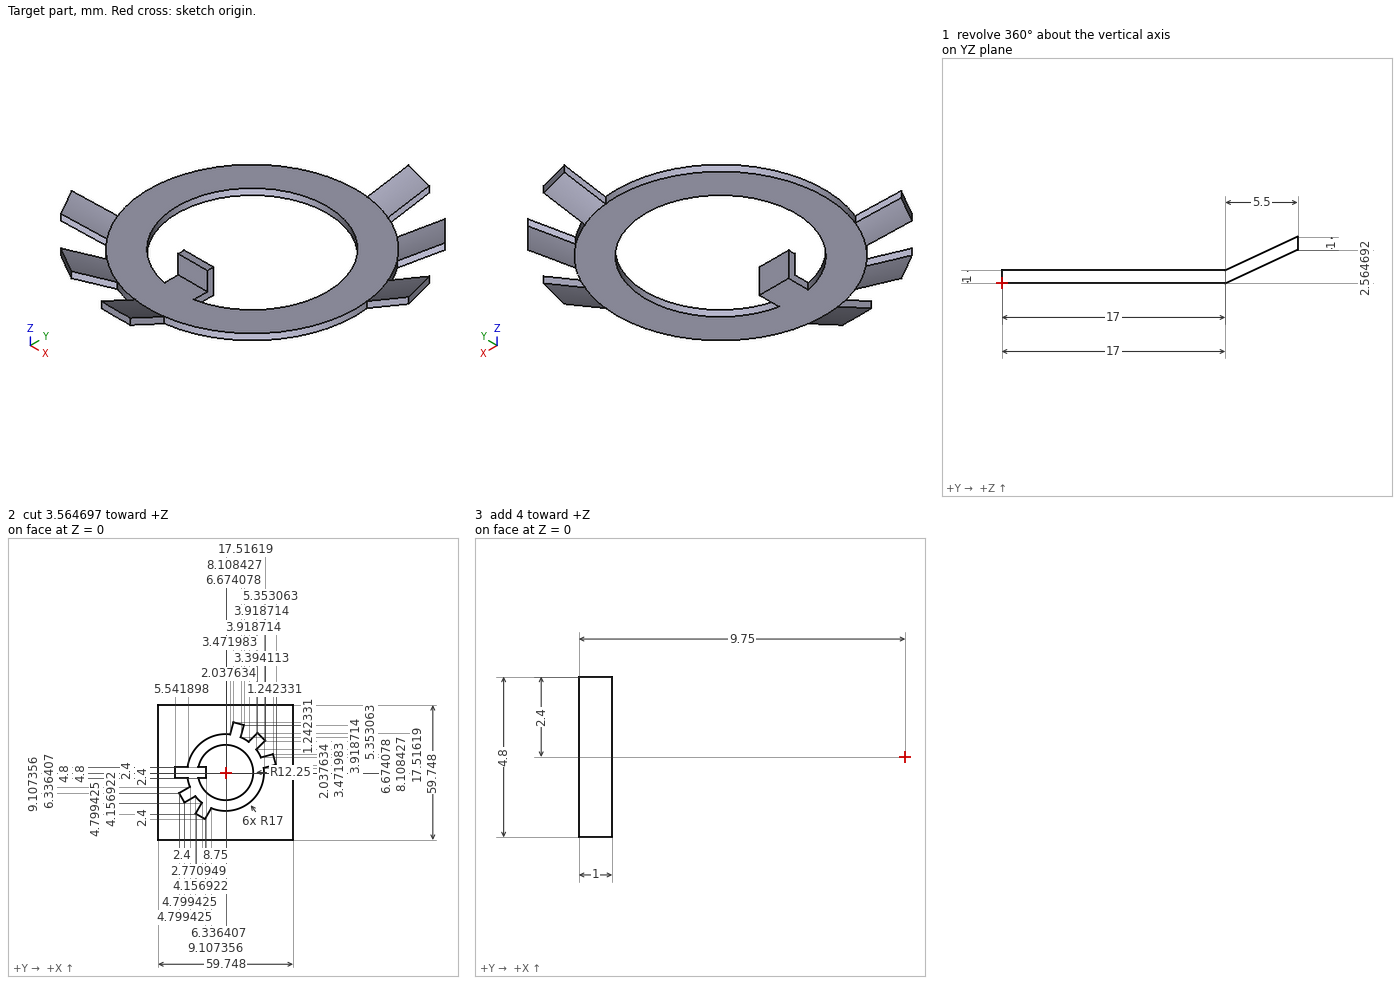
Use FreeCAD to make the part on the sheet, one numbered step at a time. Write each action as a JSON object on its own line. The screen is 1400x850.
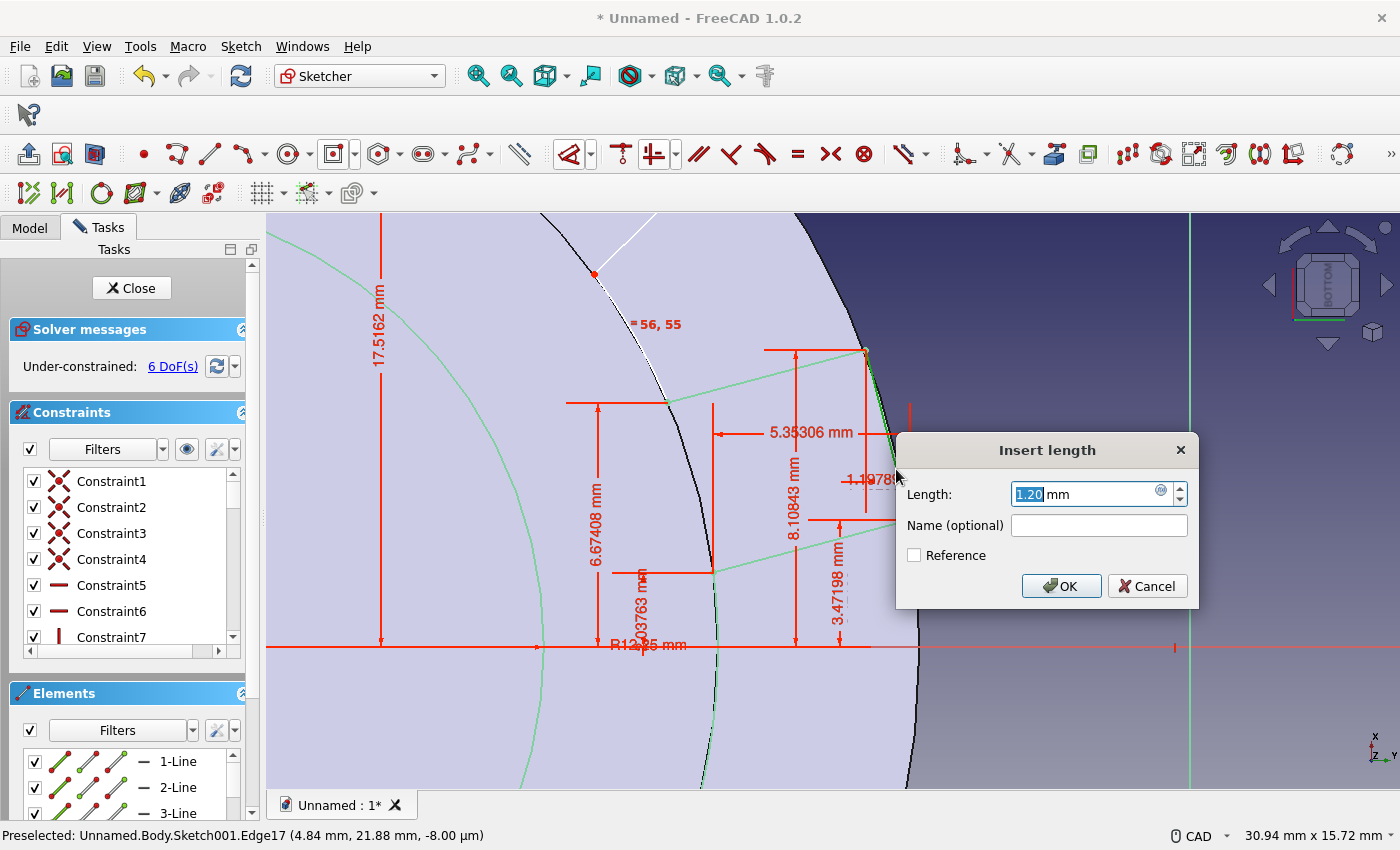
{"action": "type", "text": "1.242331"}
{"action": "key", "text": "Return"}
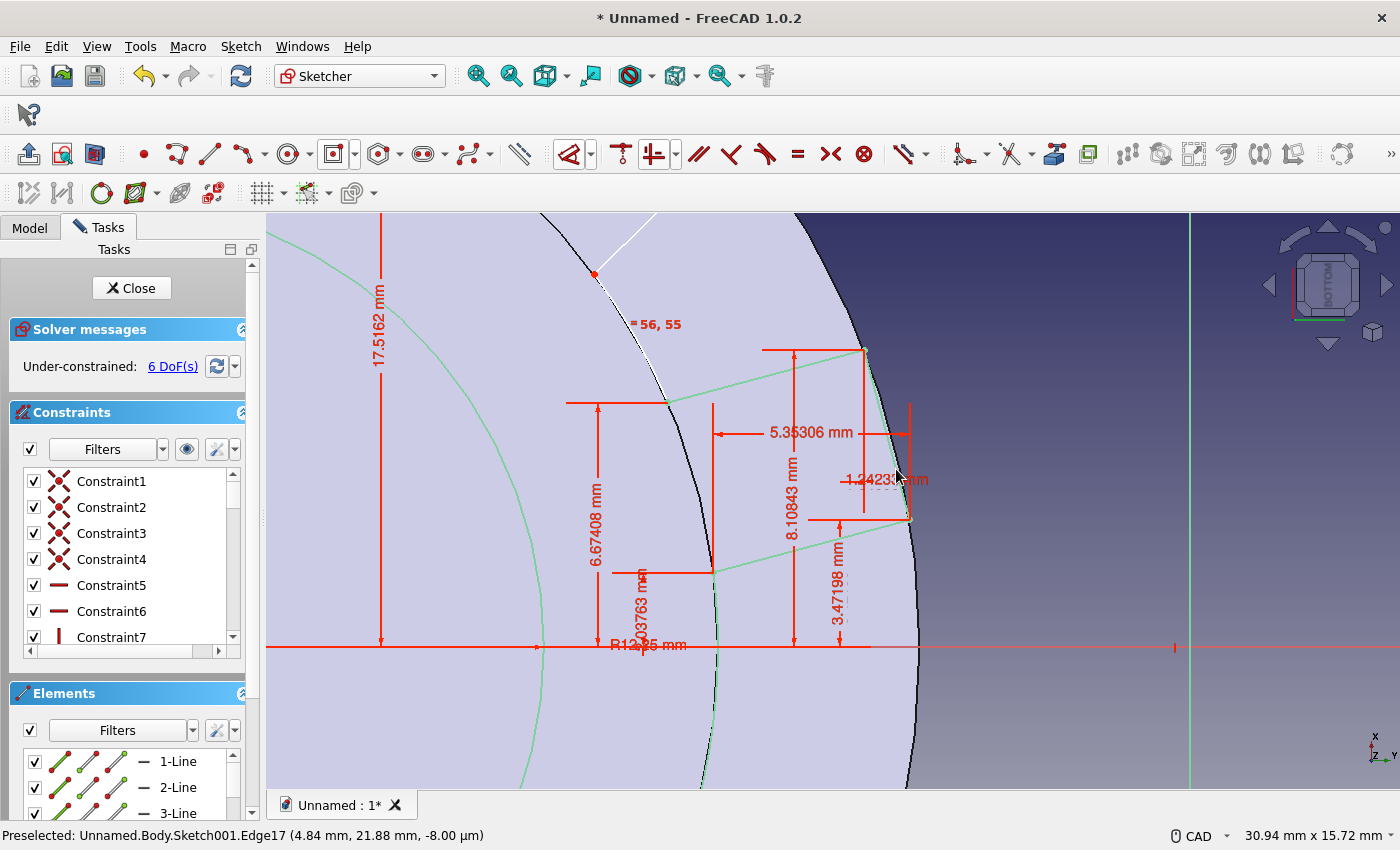
{"action": "scroll", "coordinate": [897, 472], "scroll_direction": "down", "scroll_amount": 9}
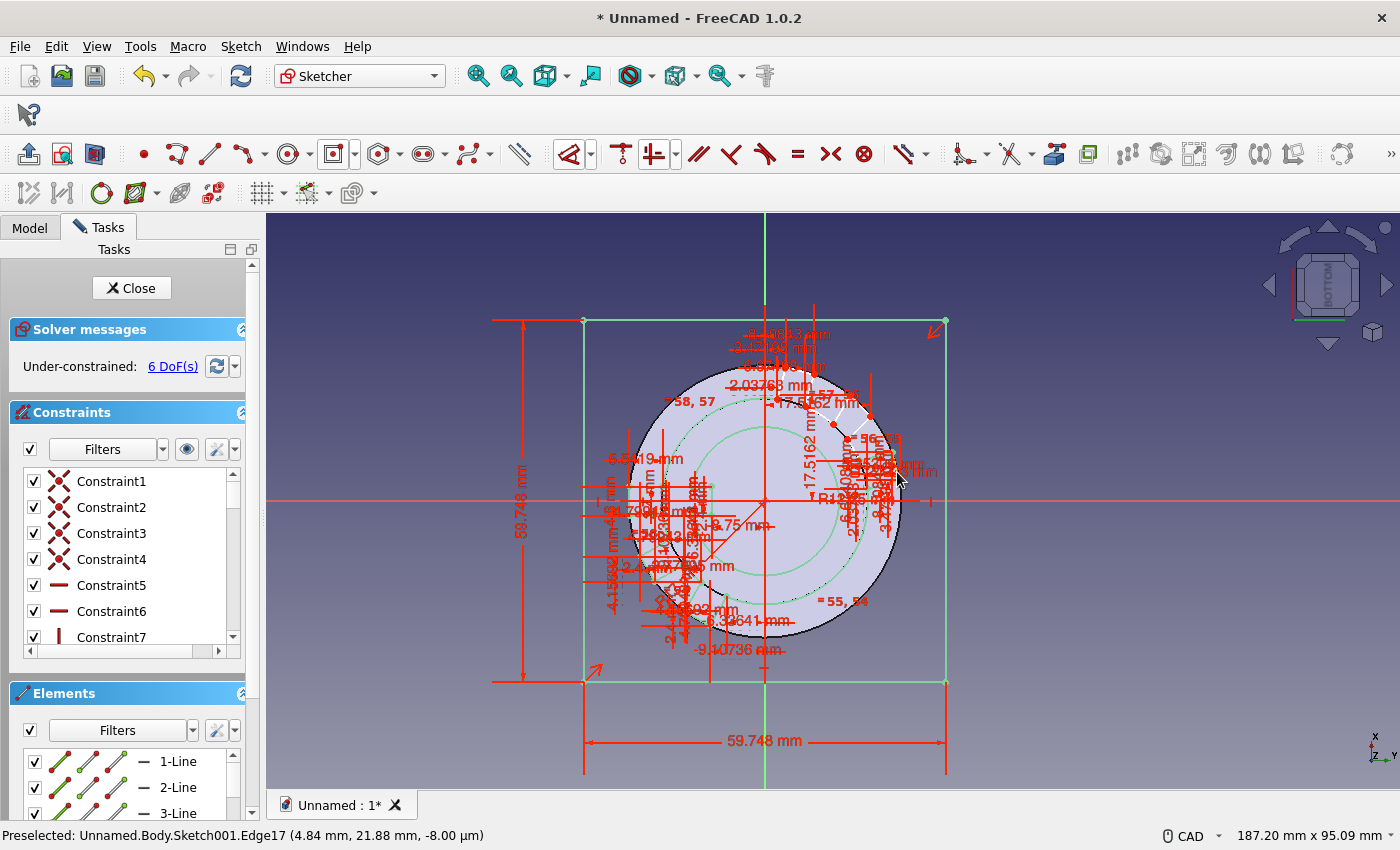
{"action": "scroll", "coordinate": [852, 435], "scroll_direction": "up", "scroll_amount": 4}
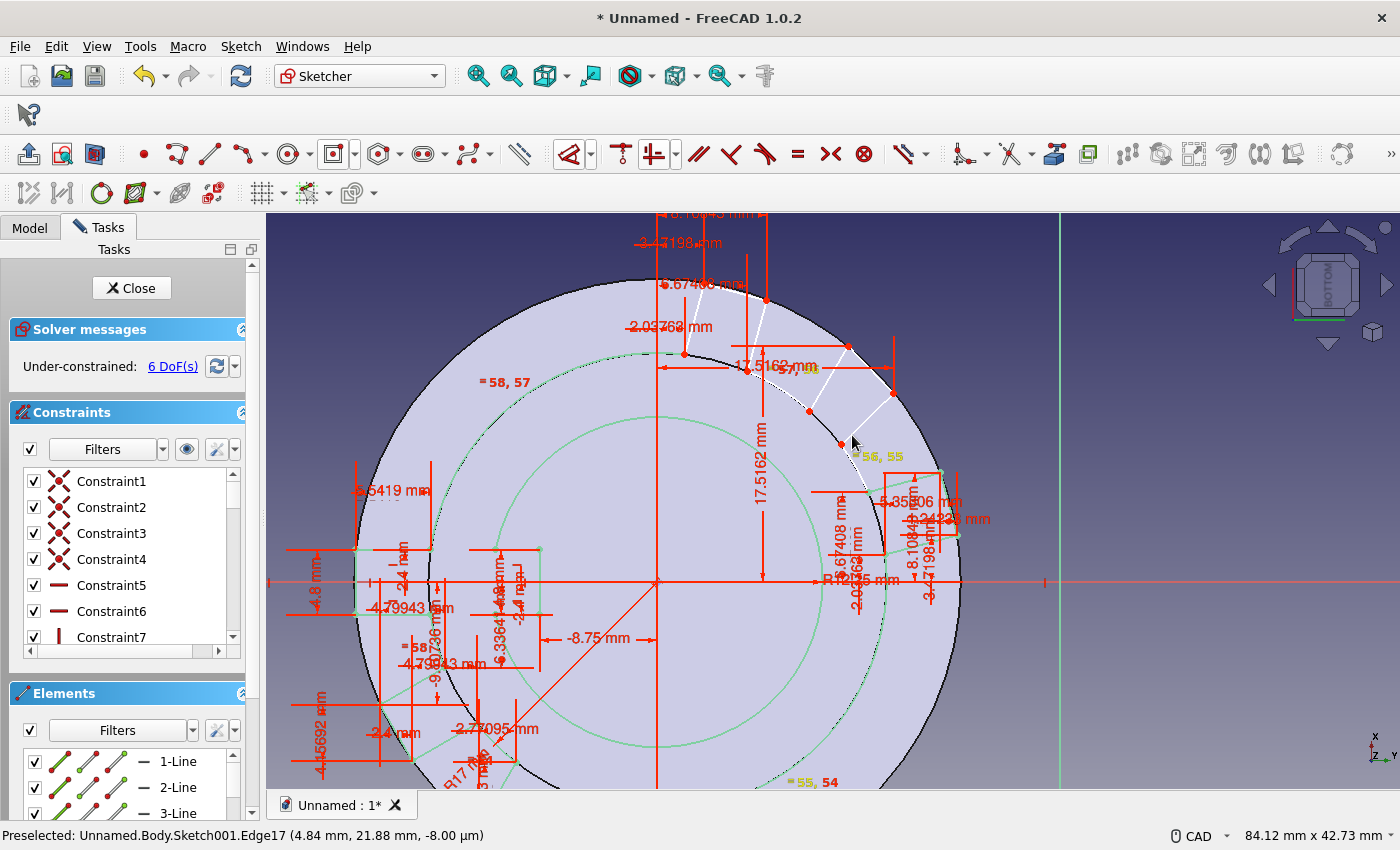
{"action": "left_click", "coordinate": [852, 435]}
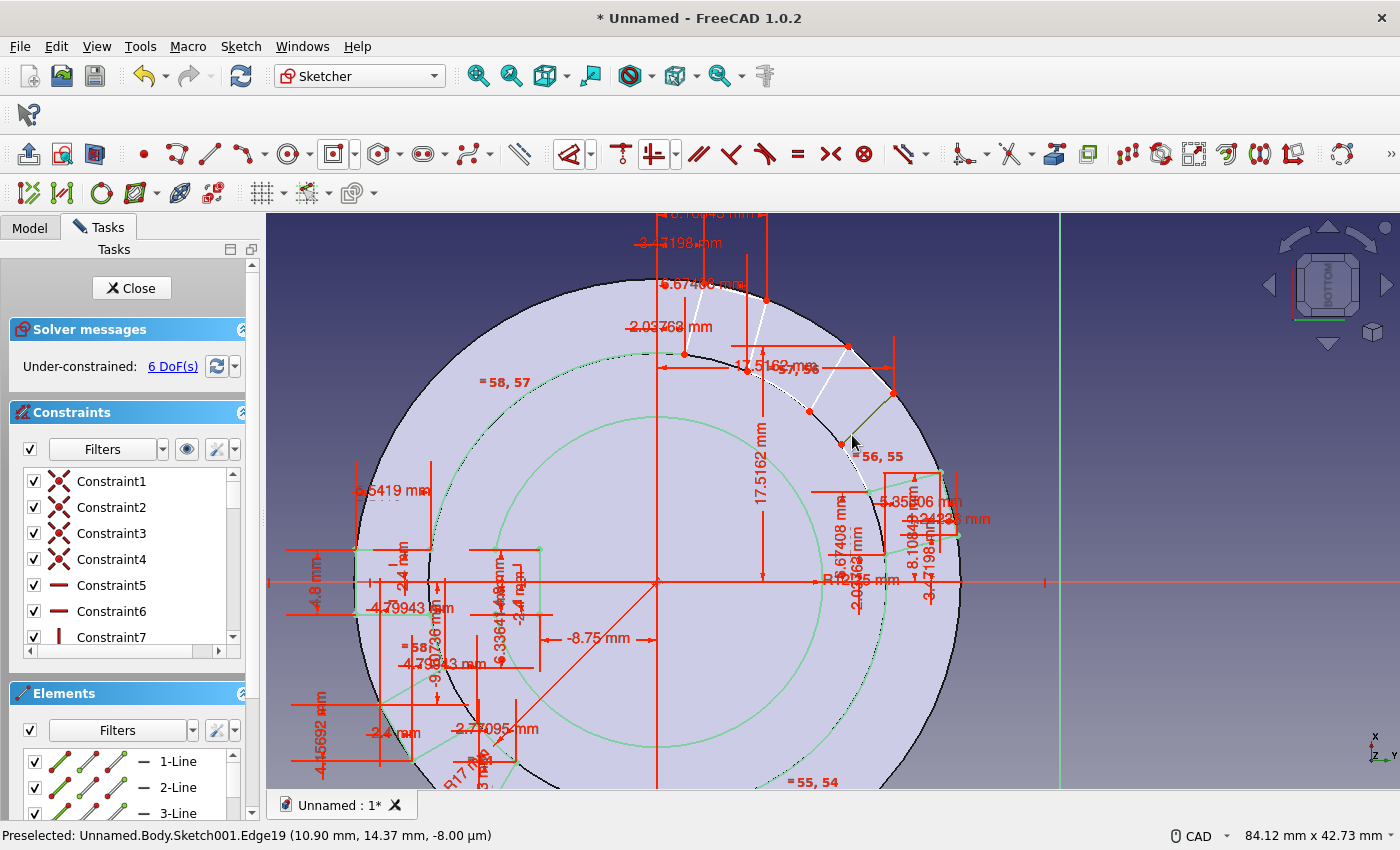
{"action": "left_click", "coordinate": [590, 154]}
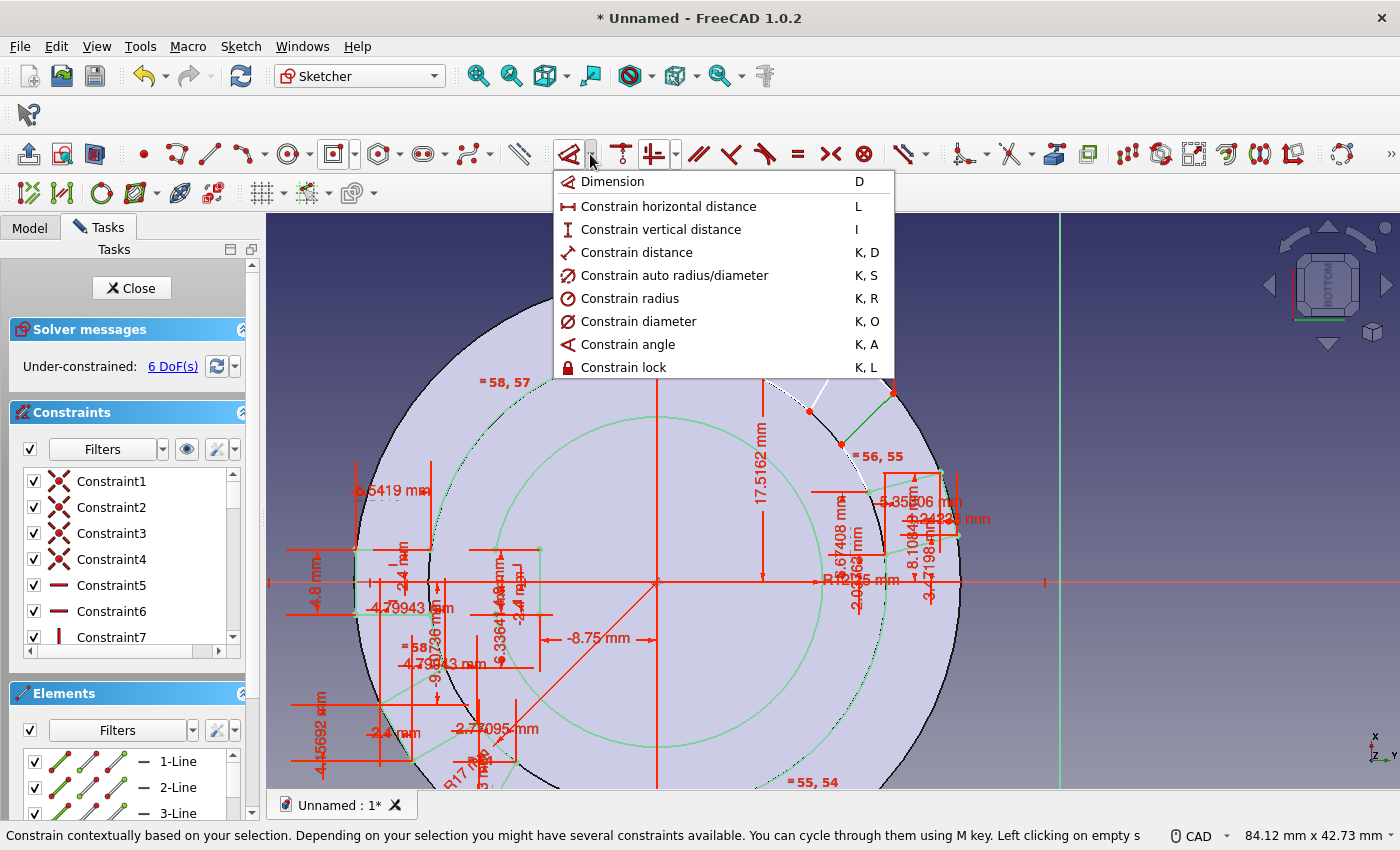
{"action": "left_click", "coordinate": [724, 206]}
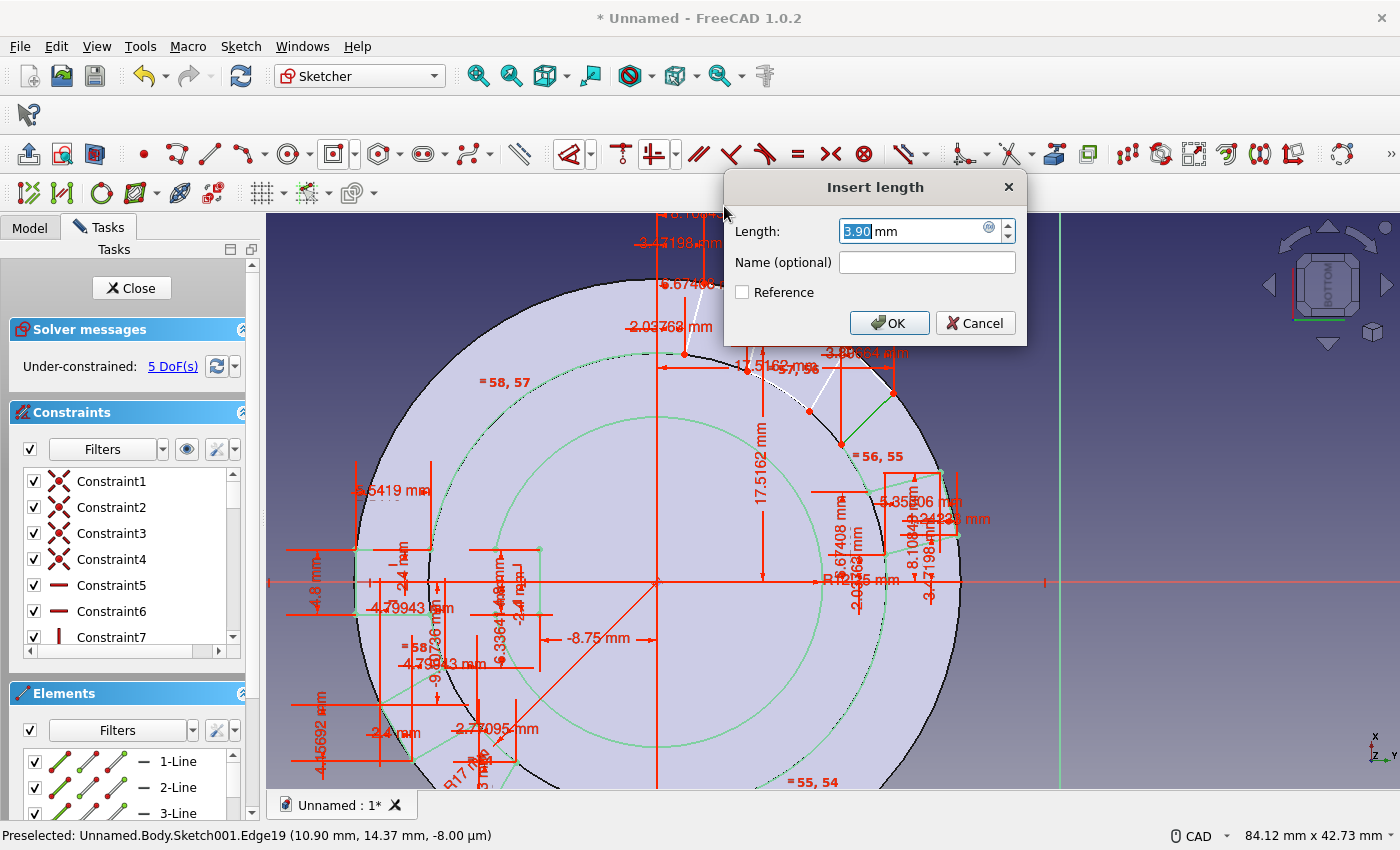
{"action": "type", "text": "3.918714"}
{"action": "key", "text": "Return"}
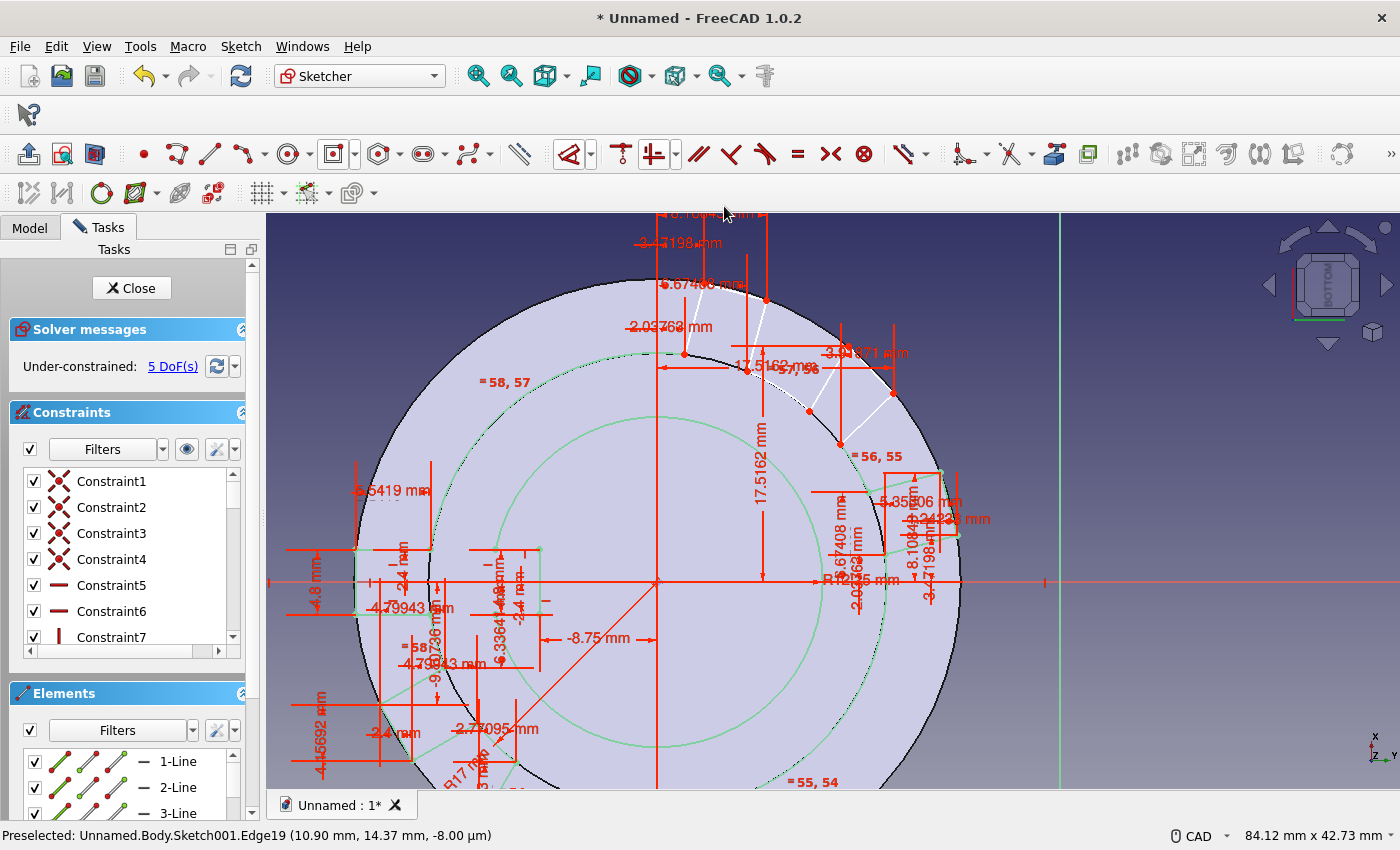
{"action": "left_click", "coordinate": [857, 429]}